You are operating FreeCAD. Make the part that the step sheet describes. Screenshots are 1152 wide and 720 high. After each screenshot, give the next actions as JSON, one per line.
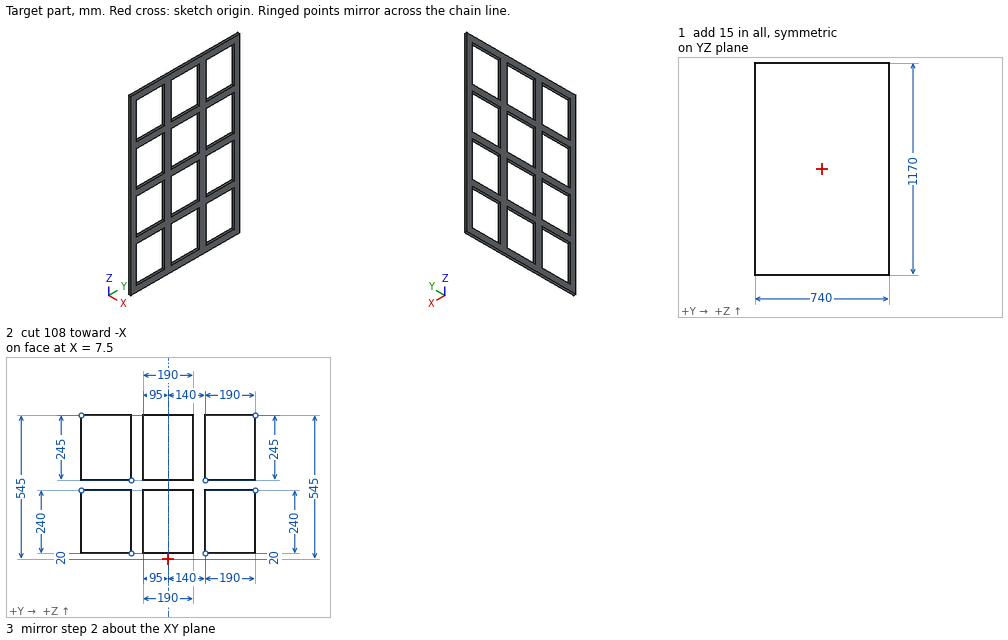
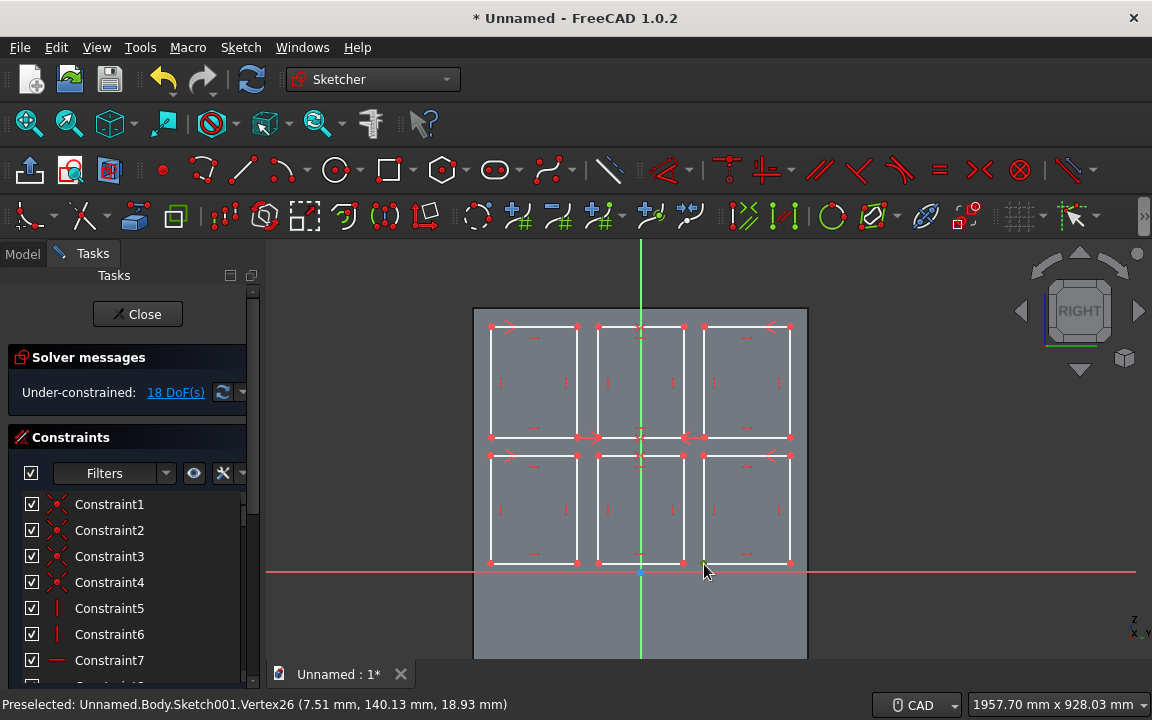
{"action": "left_click", "coordinate": [577, 564]}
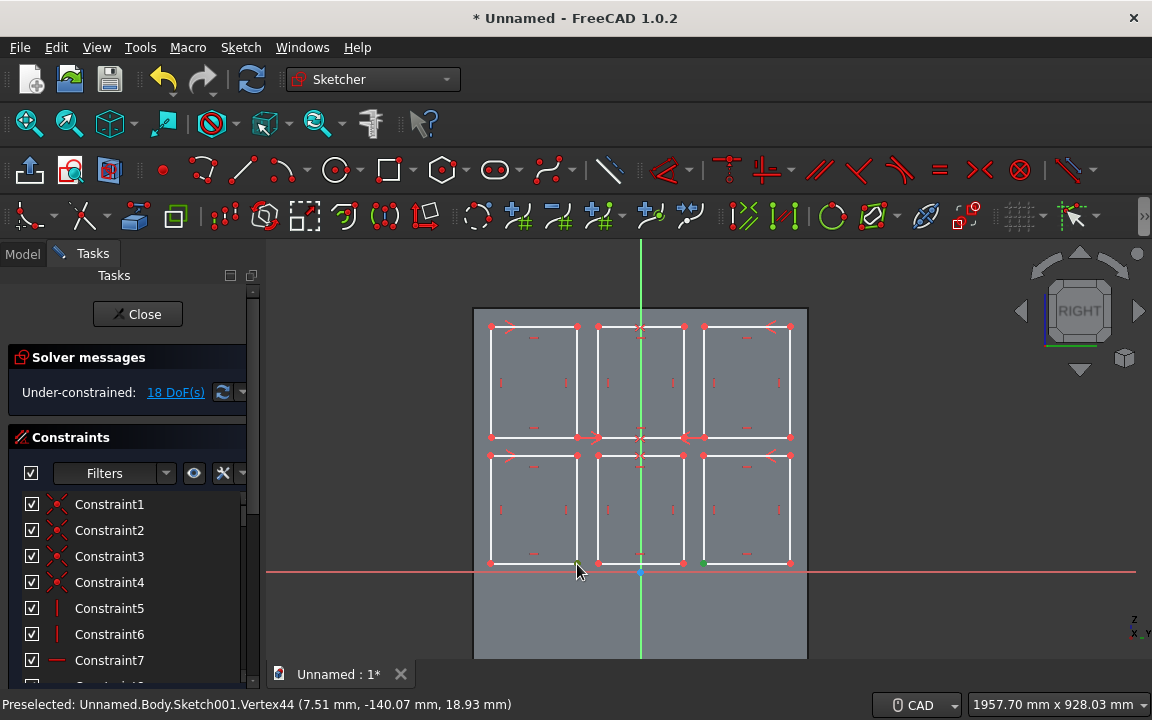
{"action": "left_click", "coordinate": [641, 605]}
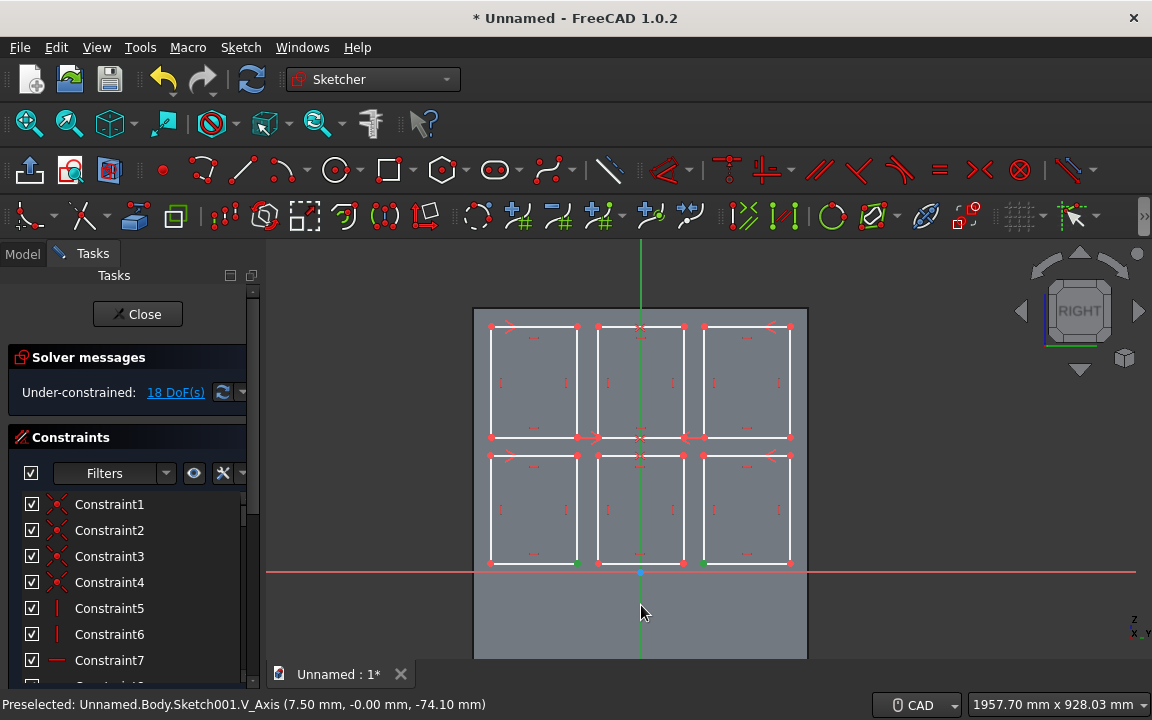
{"action": "key", "text": "s"}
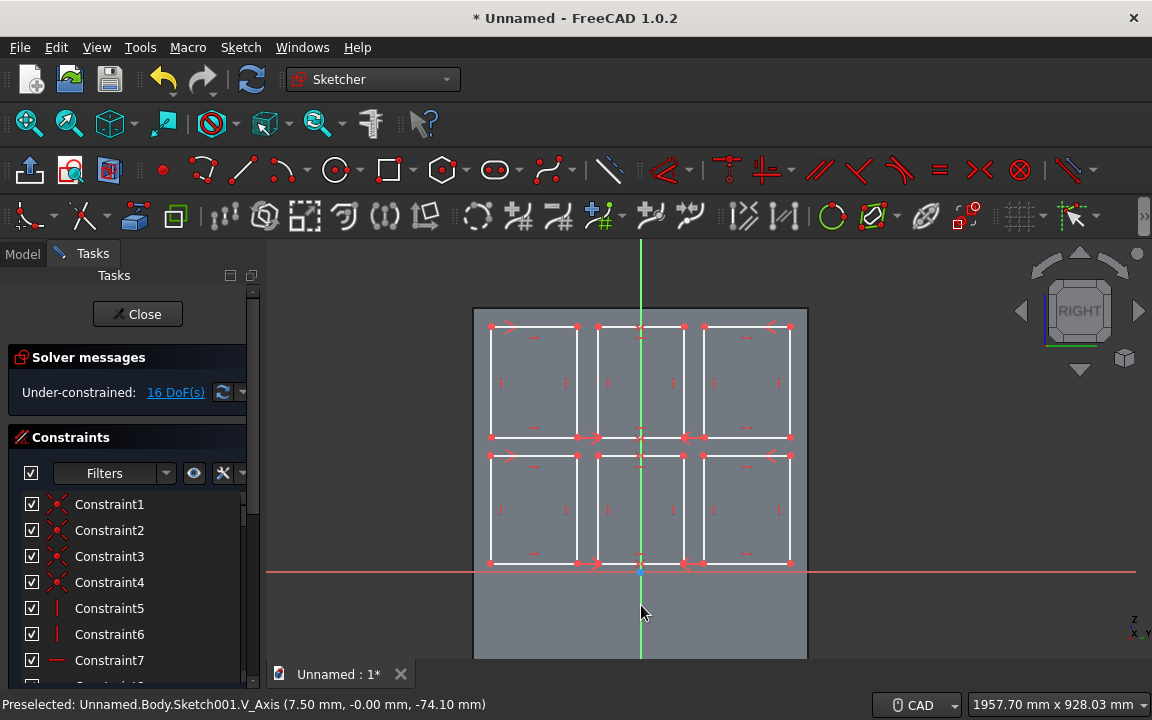
{"action": "left_click", "coordinate": [664, 170]}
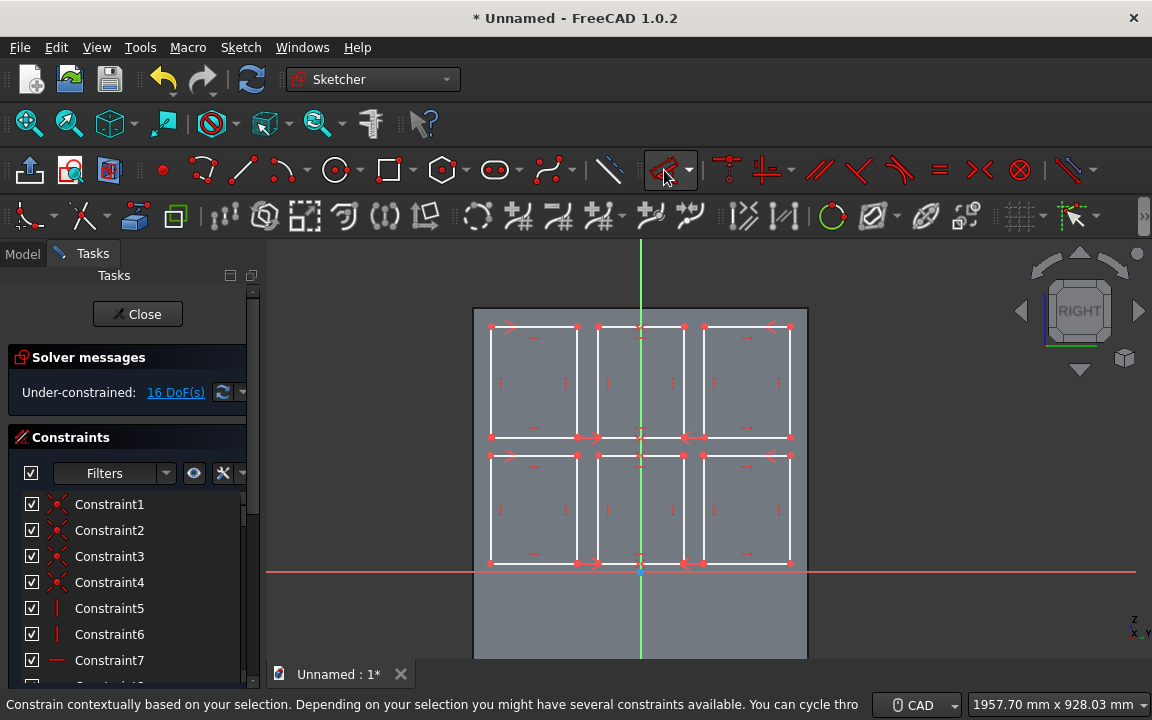
{"action": "left_click", "coordinate": [704, 360]}
{"action": "left_click", "coordinate": [738, 383]}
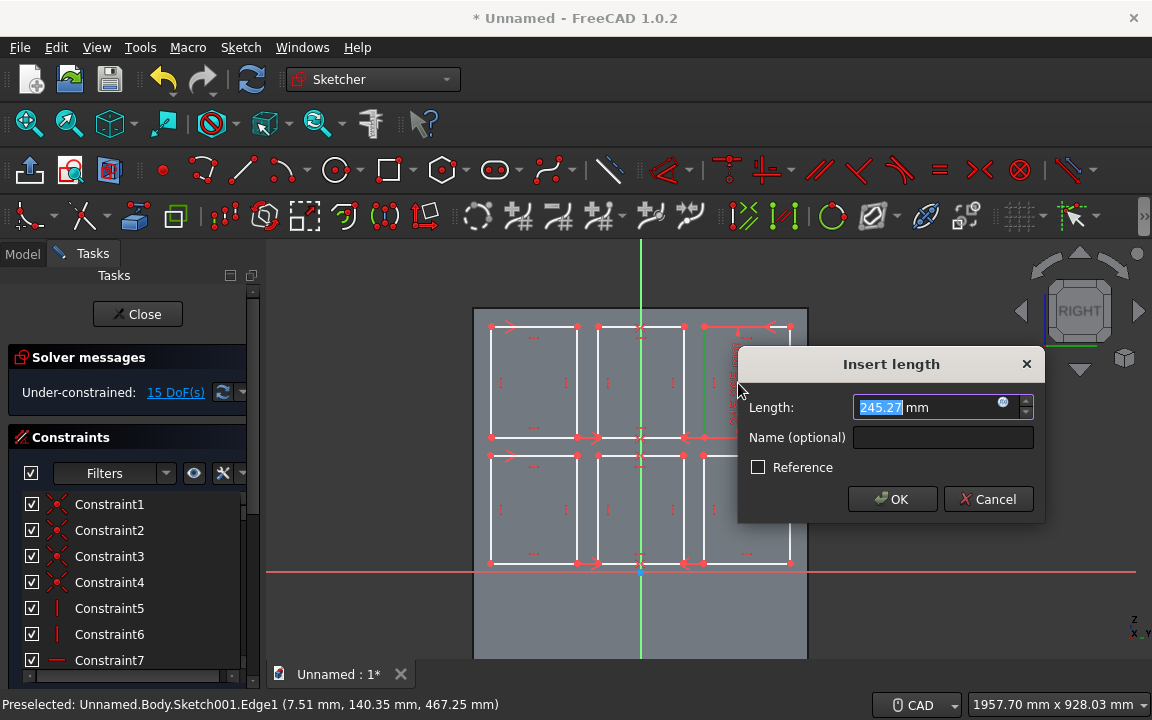
{"action": "type", "text": "245"}
{"action": "key", "text": "Return"}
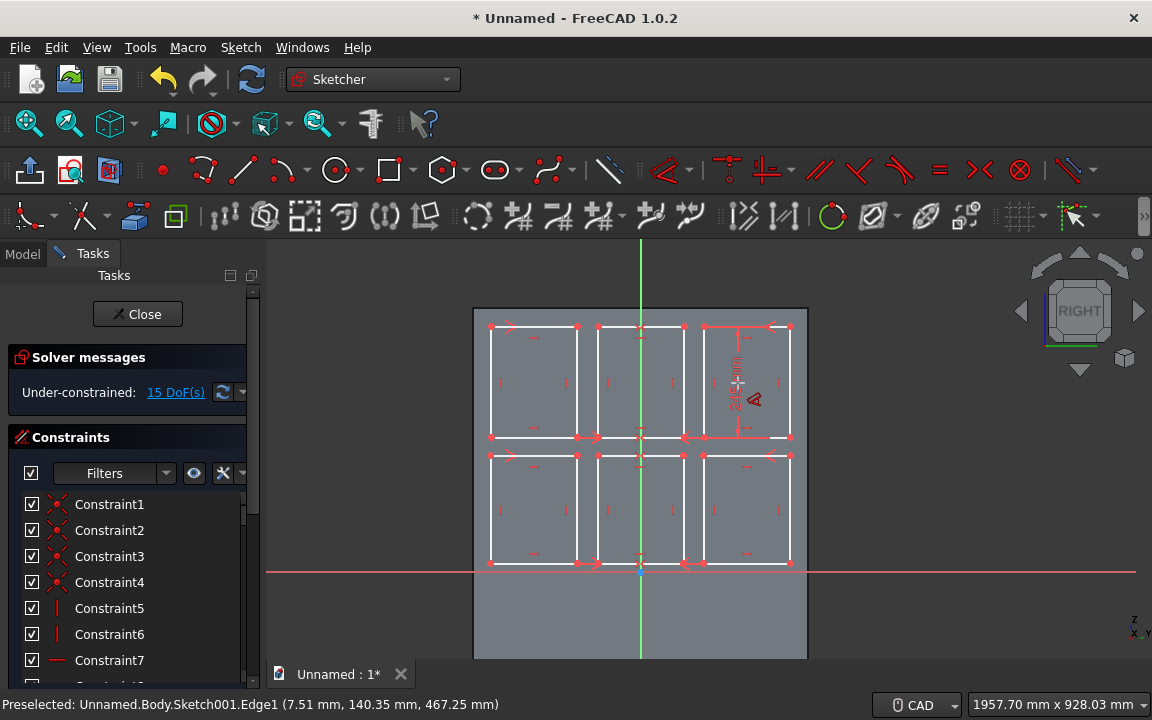
{"action": "left_click", "coordinate": [730, 438]}
{"action": "left_click", "coordinate": [747, 404]}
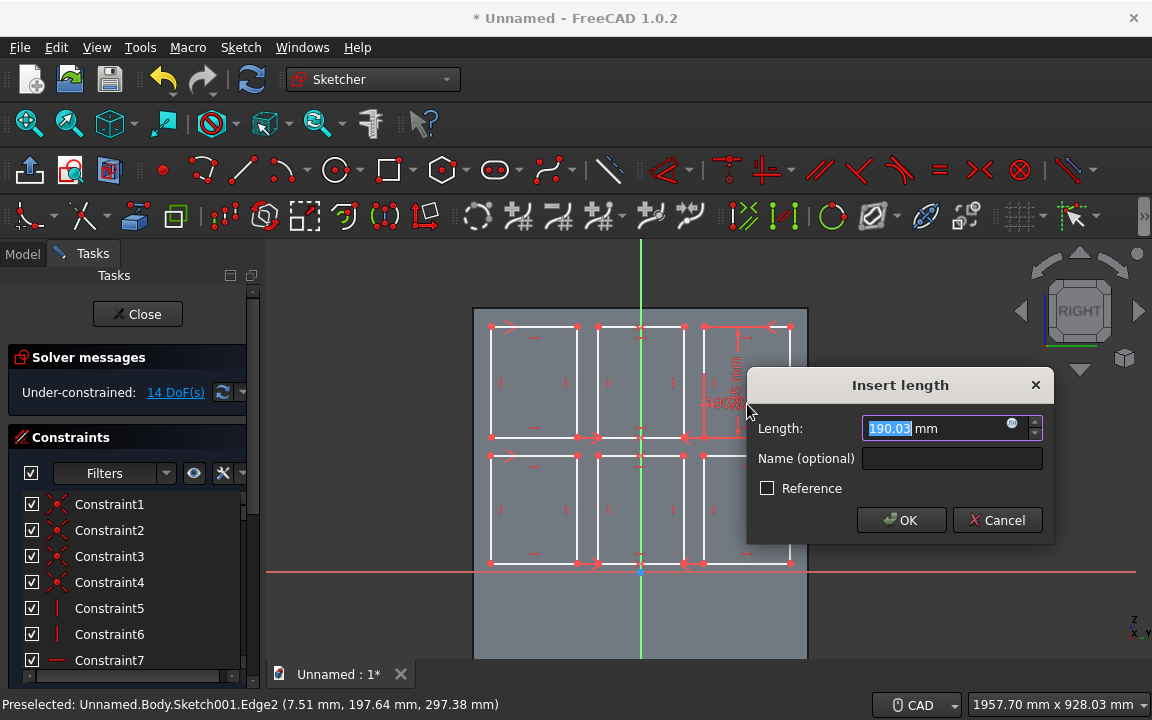
{"action": "type", "text": "190"}
{"action": "key", "text": "Return"}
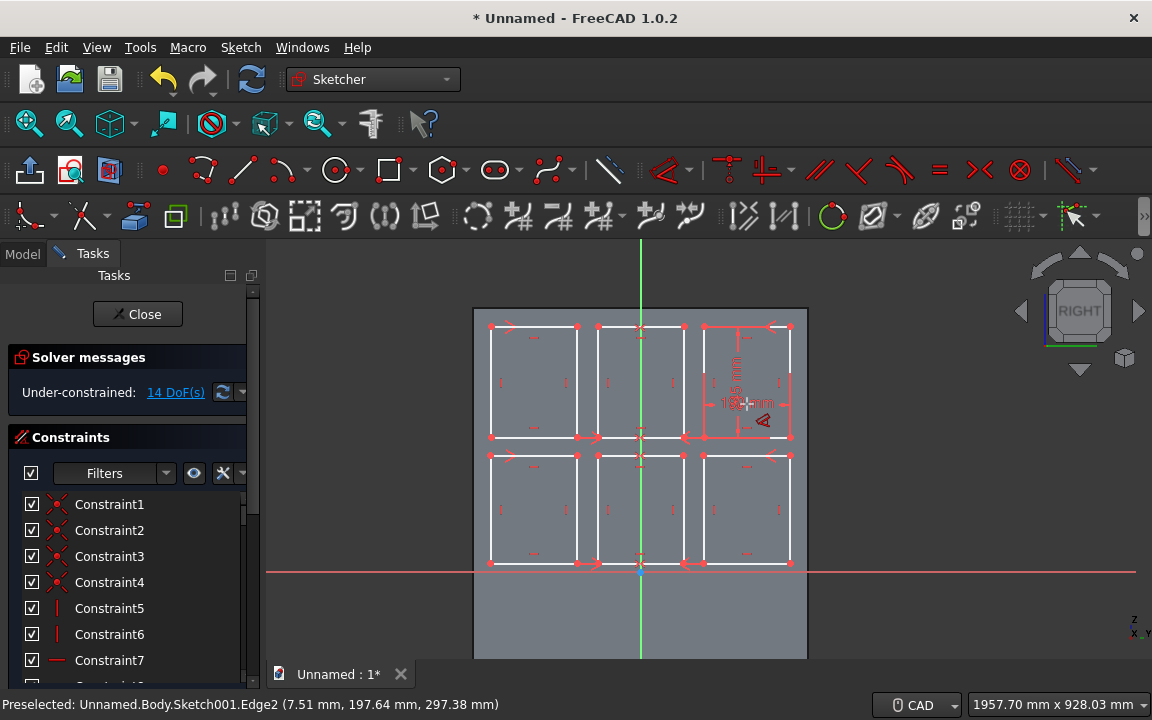
{"action": "left_click", "coordinate": [598, 360]}
{"action": "left_click", "coordinate": [564, 383]}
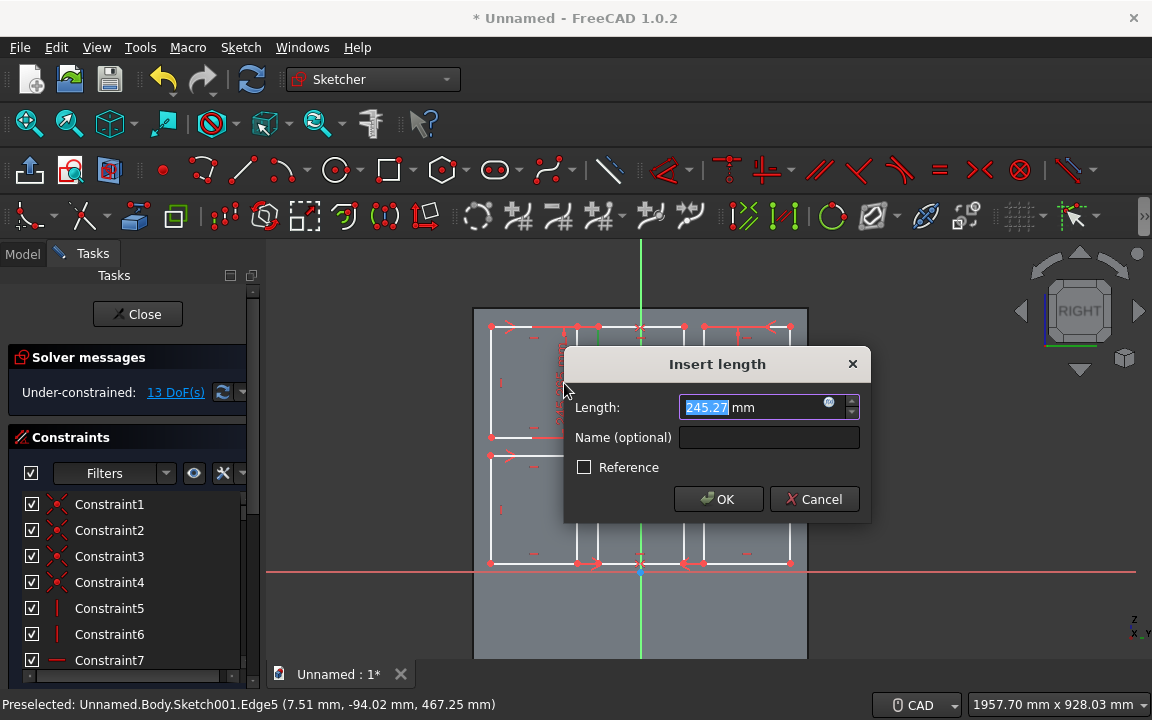
{"action": "type", "text": "245"}
{"action": "key", "text": "Return"}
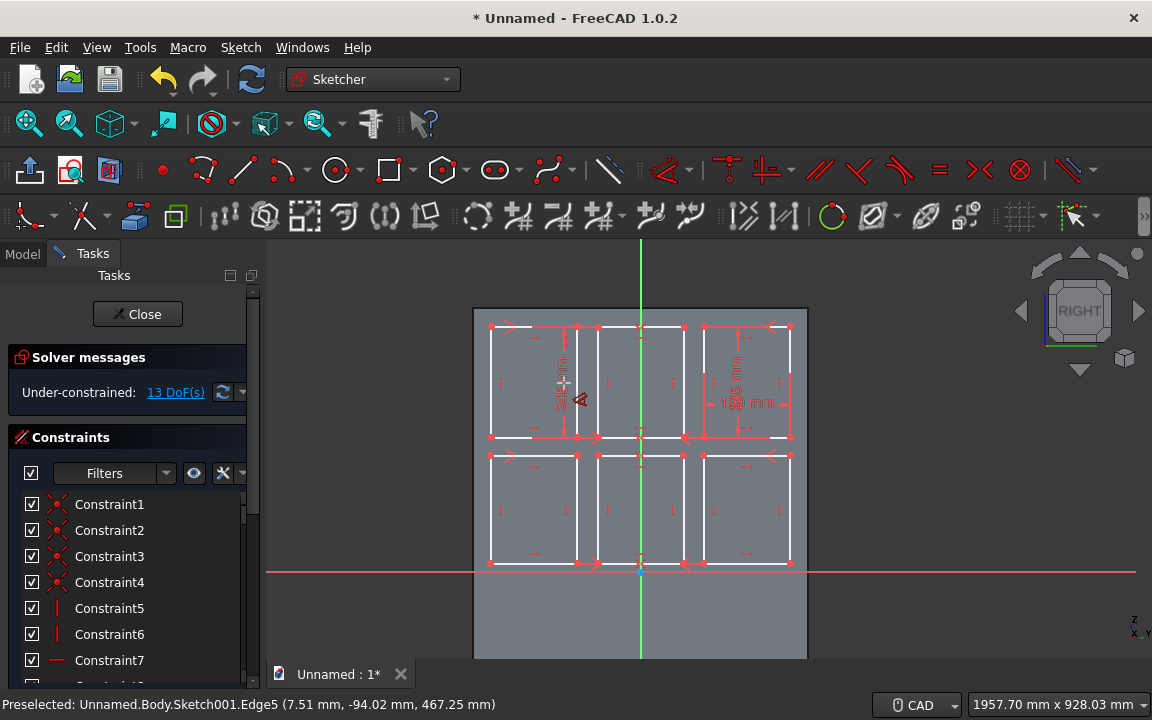
{"action": "left_click", "coordinate": [624, 438]}
{"action": "left_click", "coordinate": [621, 404]}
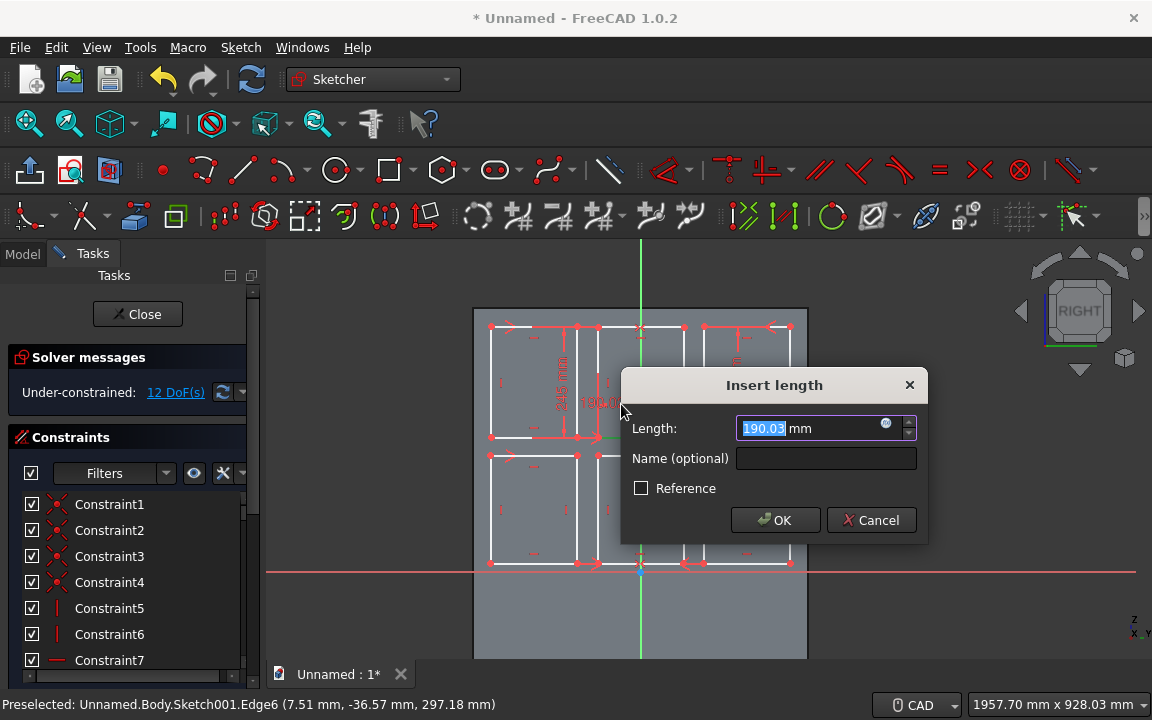
{"action": "type", "text": "190"}
{"action": "key", "text": "Return"}